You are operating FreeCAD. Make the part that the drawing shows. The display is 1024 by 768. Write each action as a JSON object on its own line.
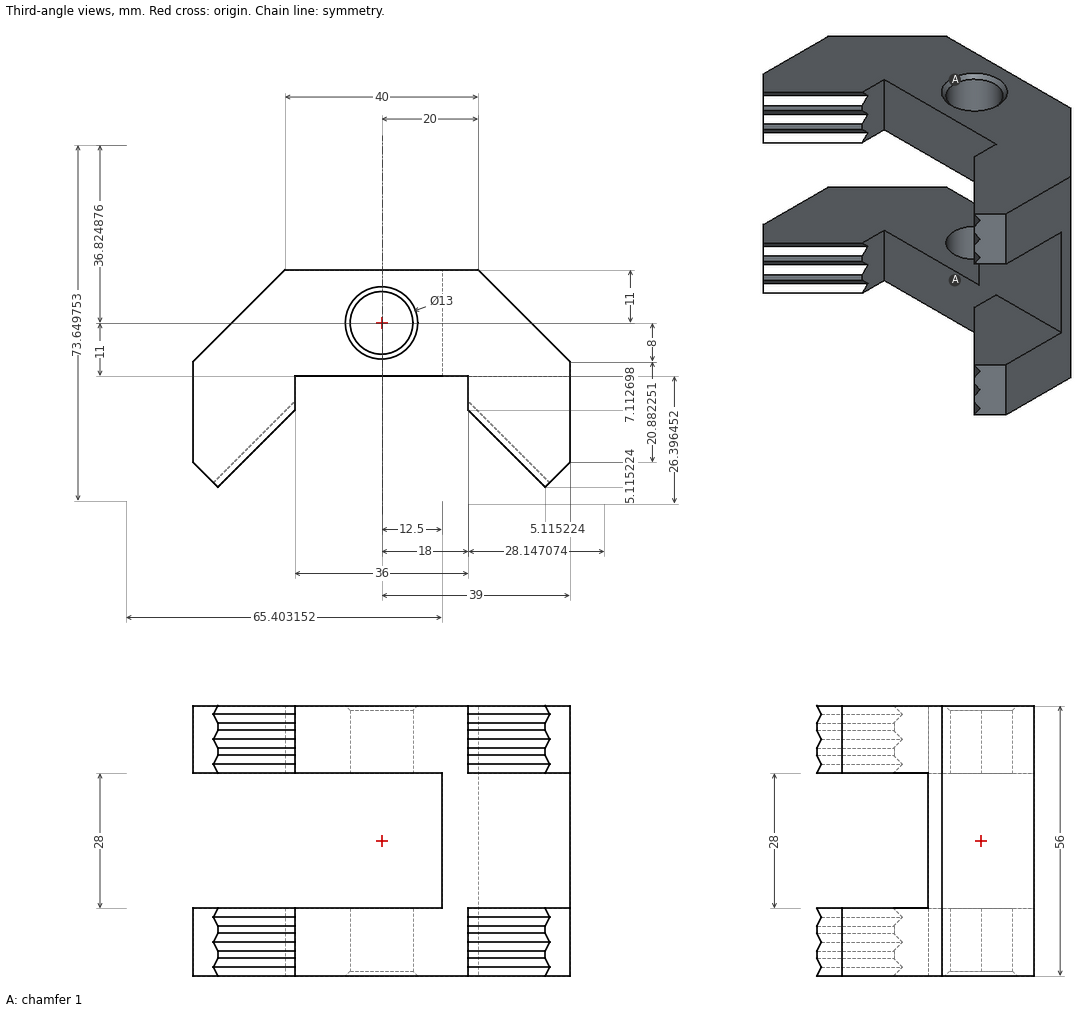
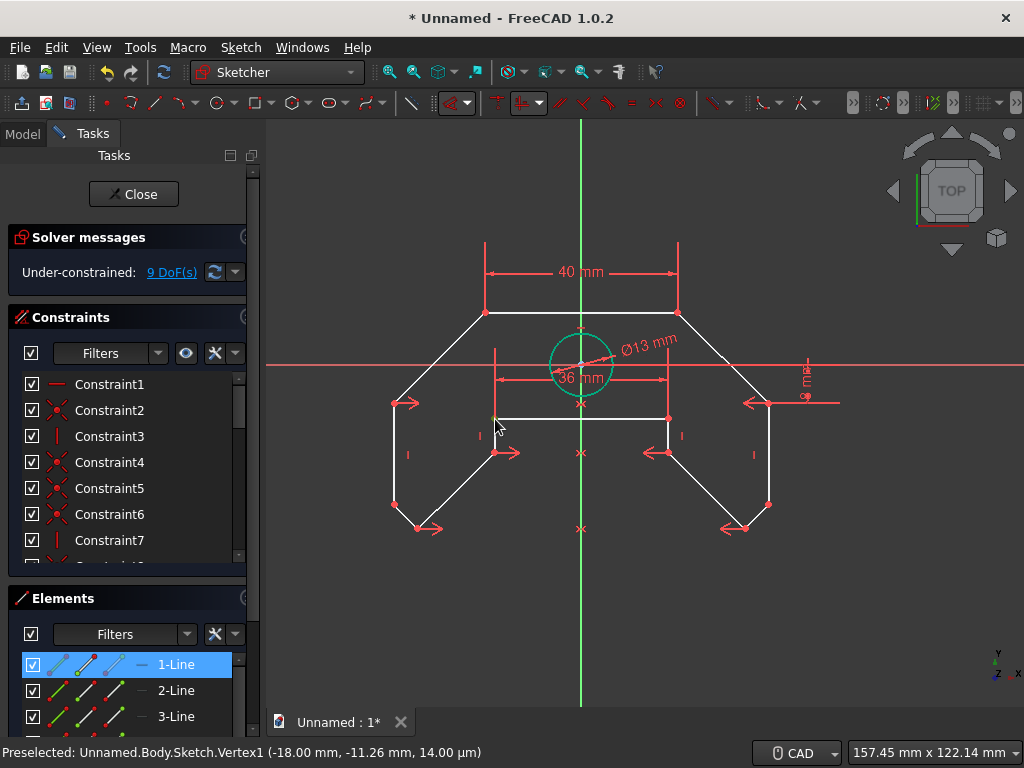
{"action": "key", "text": "i"}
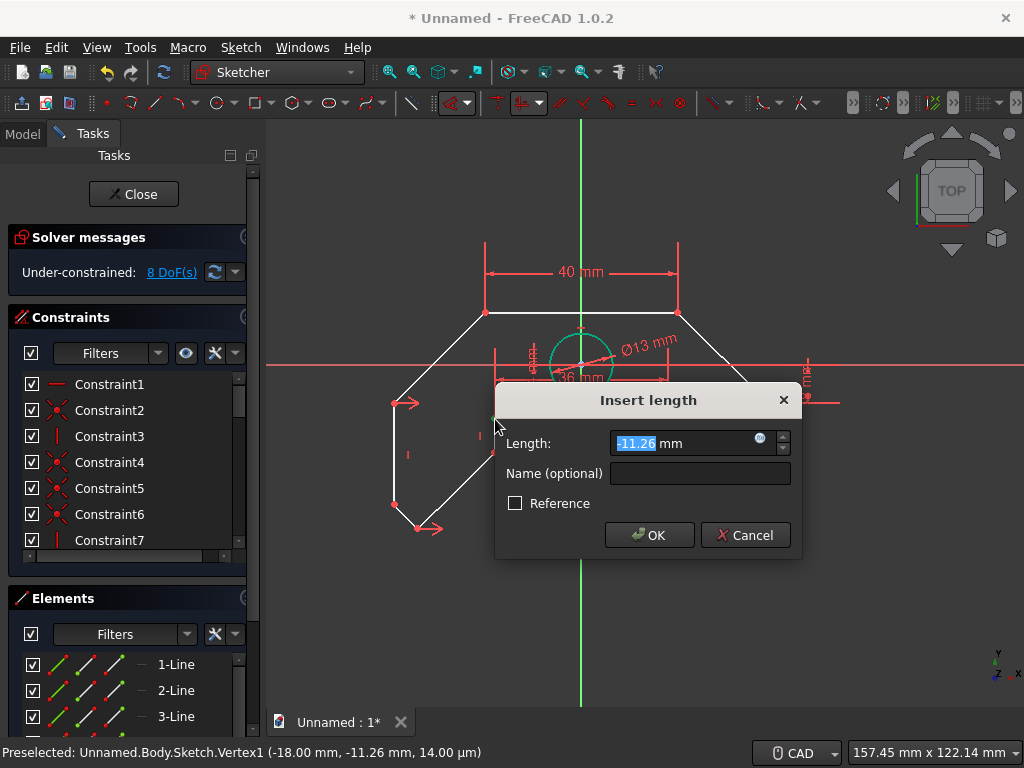
{"action": "type", "text": "-11"}
{"action": "key", "text": "Return"}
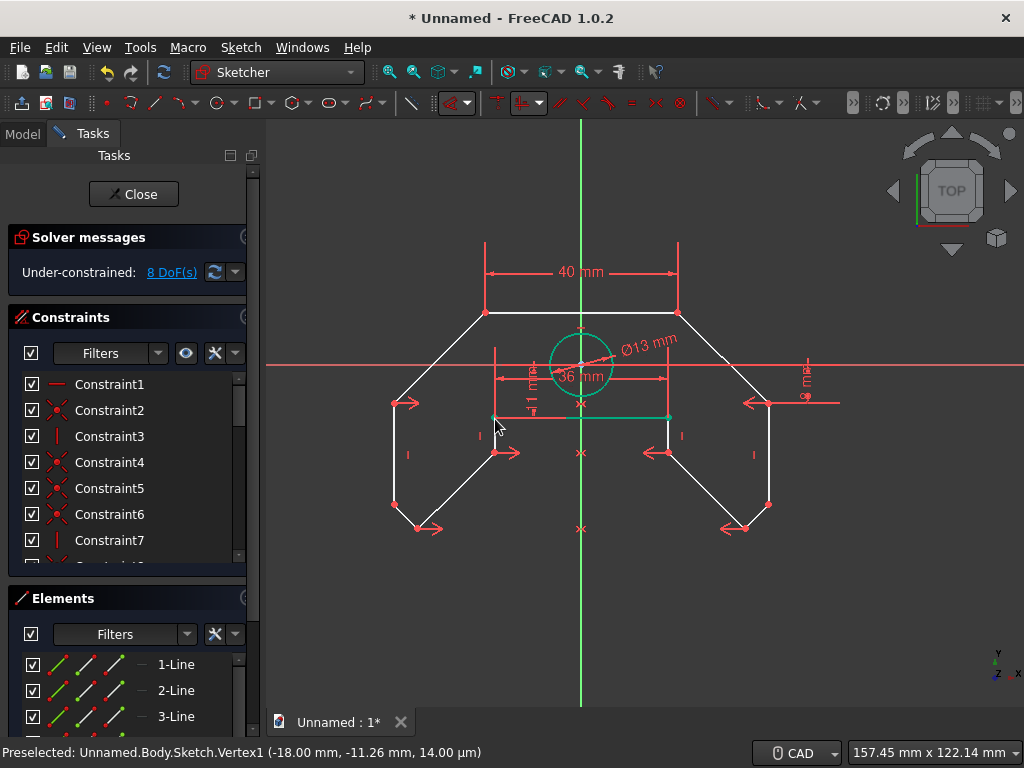
{"action": "left_click", "coordinate": [769, 505]}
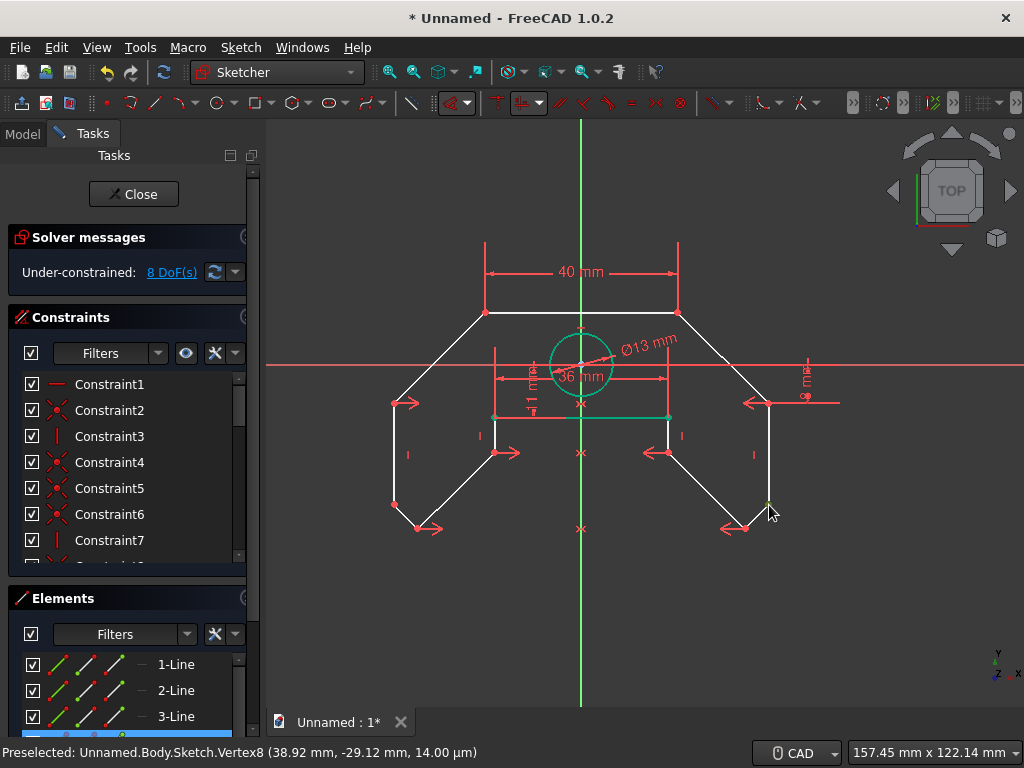
{"action": "key", "text": "l"}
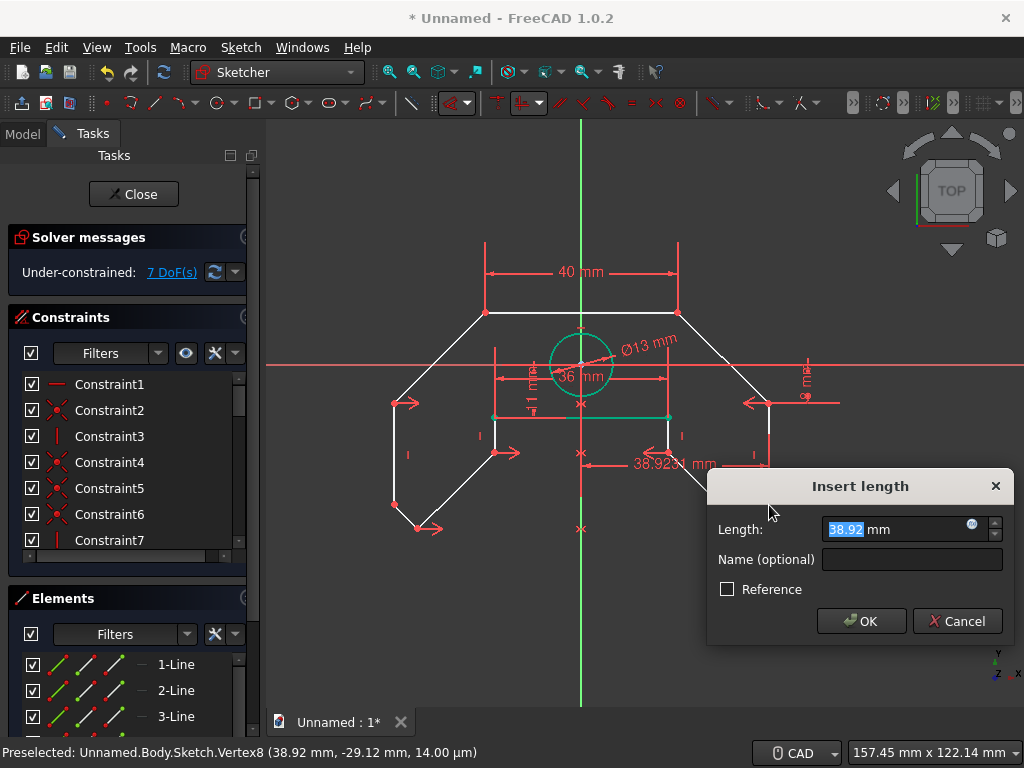
{"action": "type", "text": "39"}
{"action": "key", "text": "Return"}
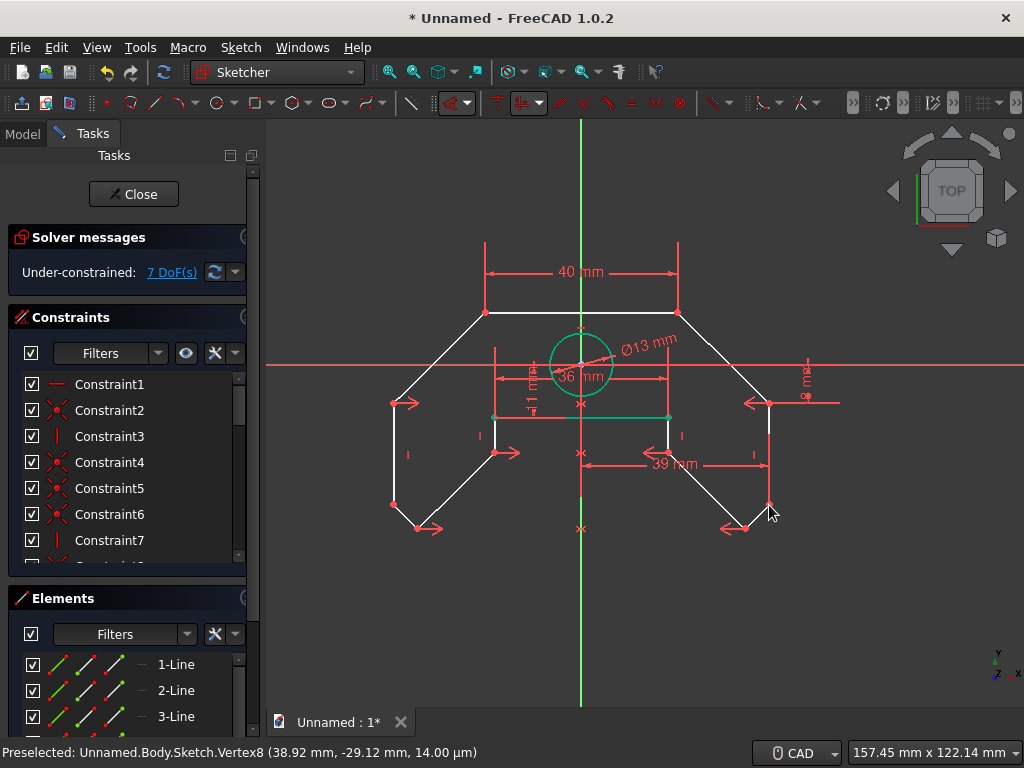
{"action": "left_click", "coordinate": [678, 313]}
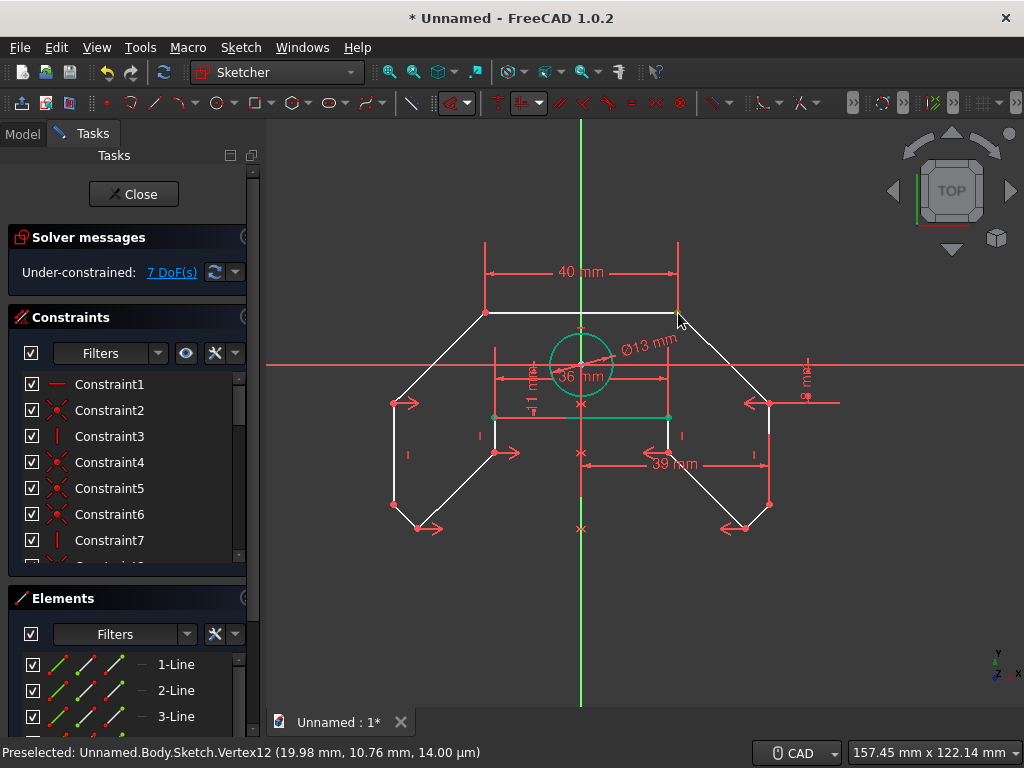
{"action": "key", "text": "l"}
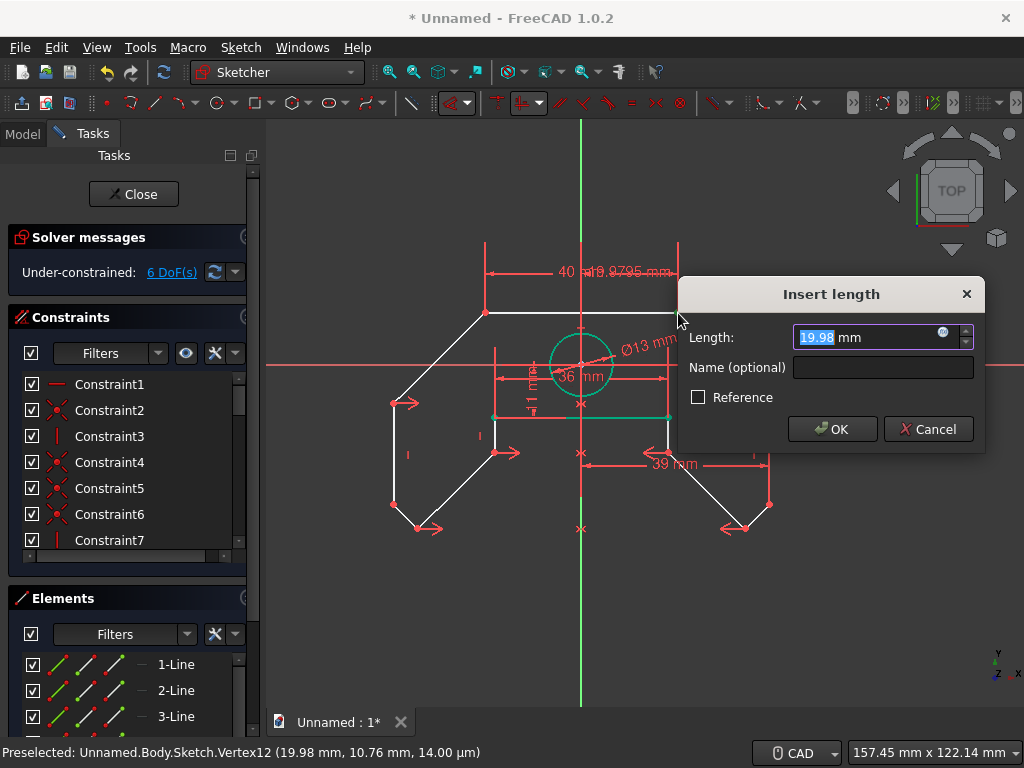
{"action": "type", "text": "20"}
{"action": "key", "text": "Return"}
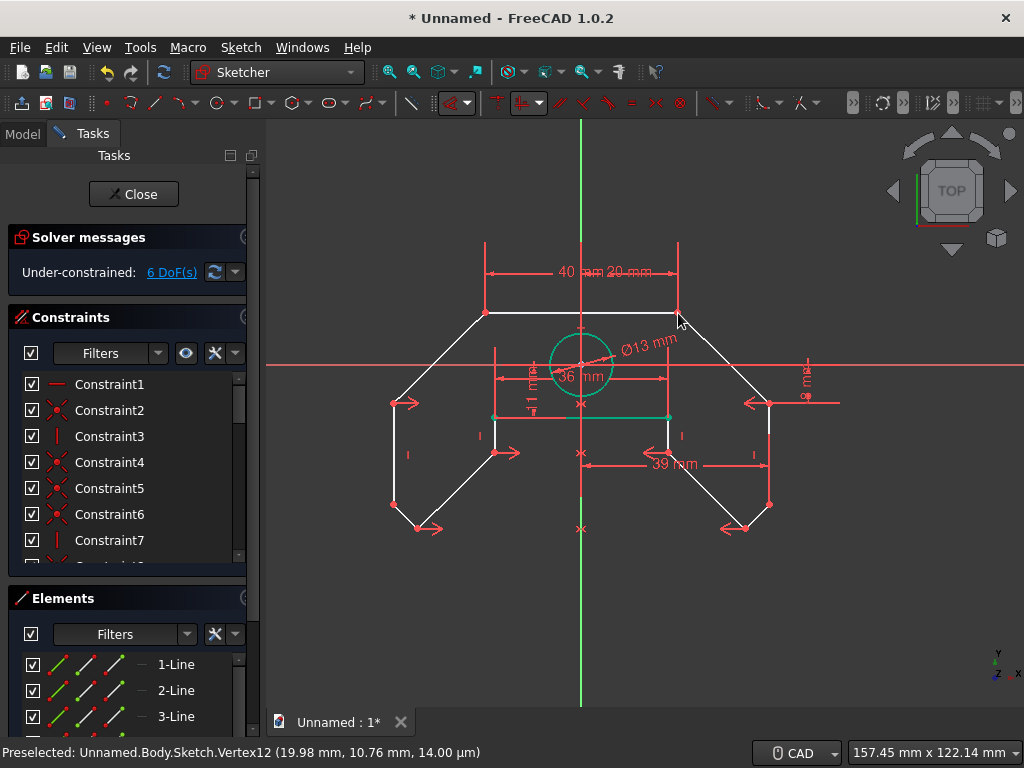
{"action": "left_click", "coordinate": [678, 313]}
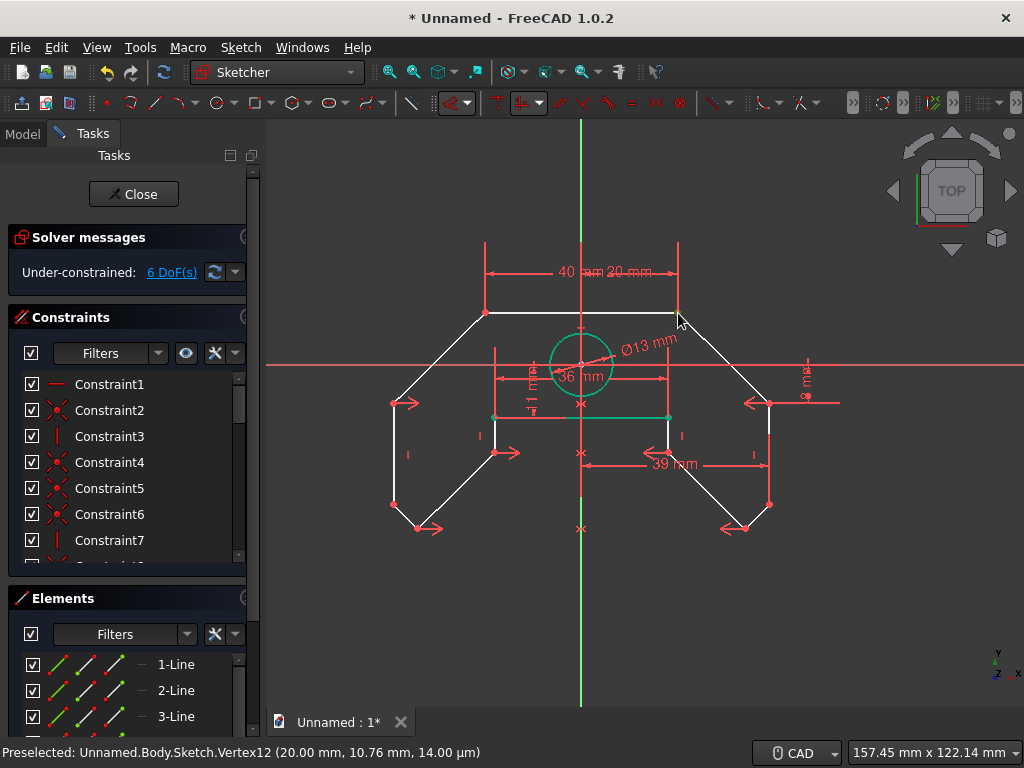
{"action": "key", "text": "i"}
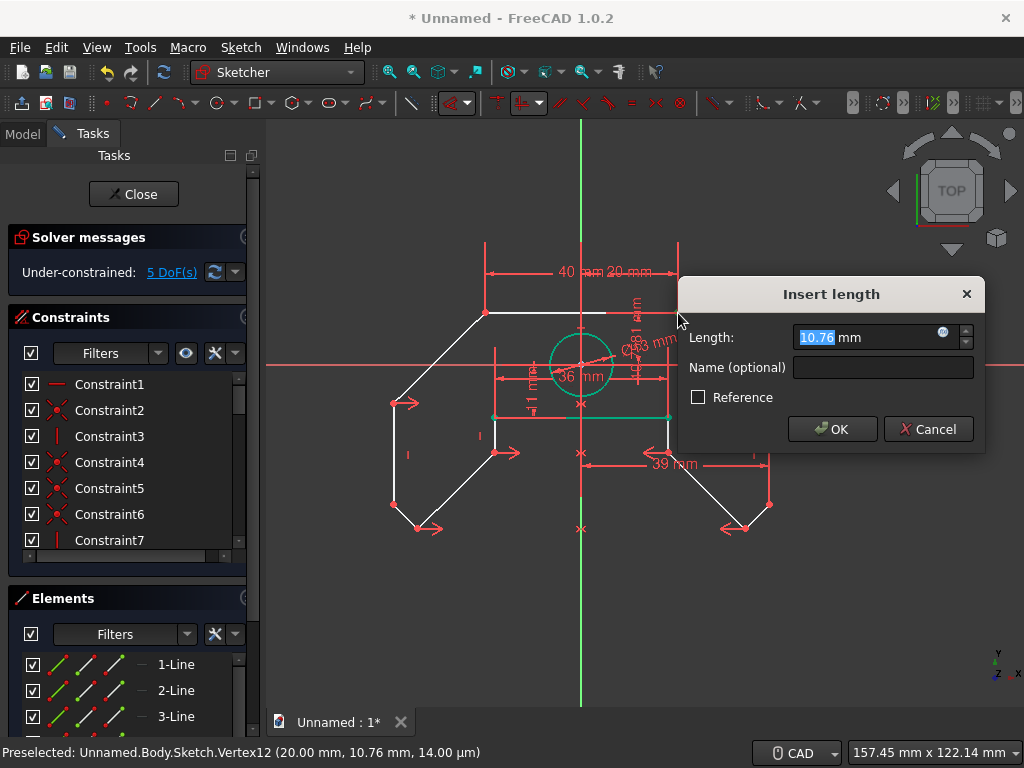
{"action": "type", "text": "11"}
{"action": "key", "text": "Return"}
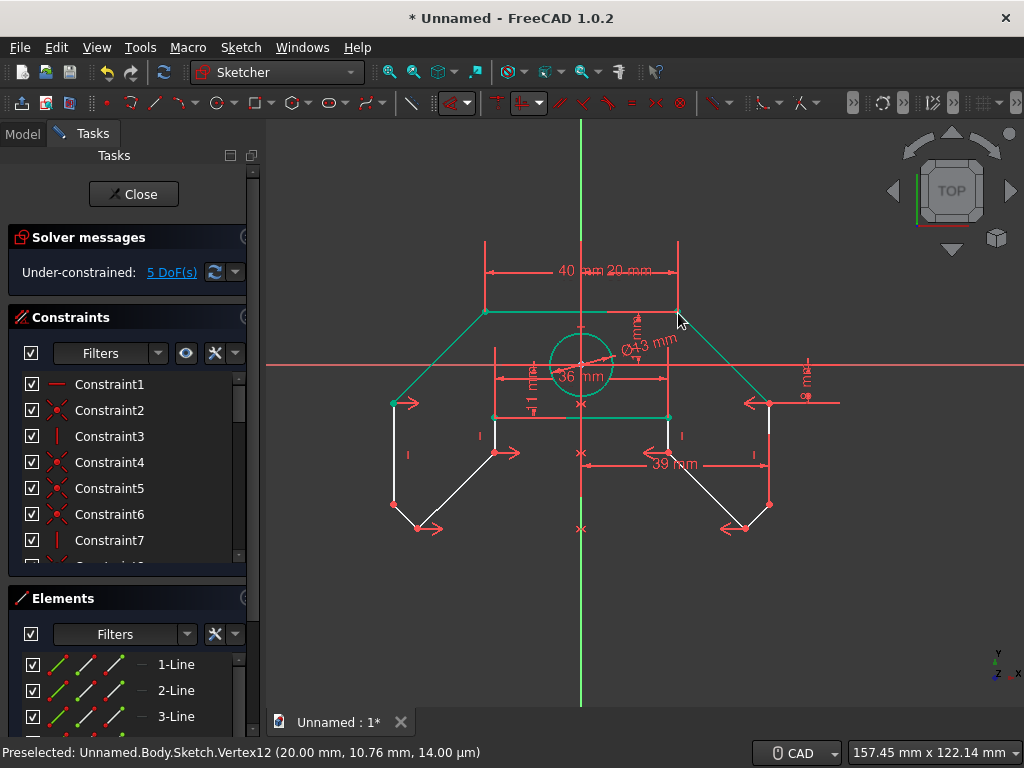
{"action": "scroll", "coordinate": [668, 428], "scroll_direction": "up", "scroll_amount": 2}